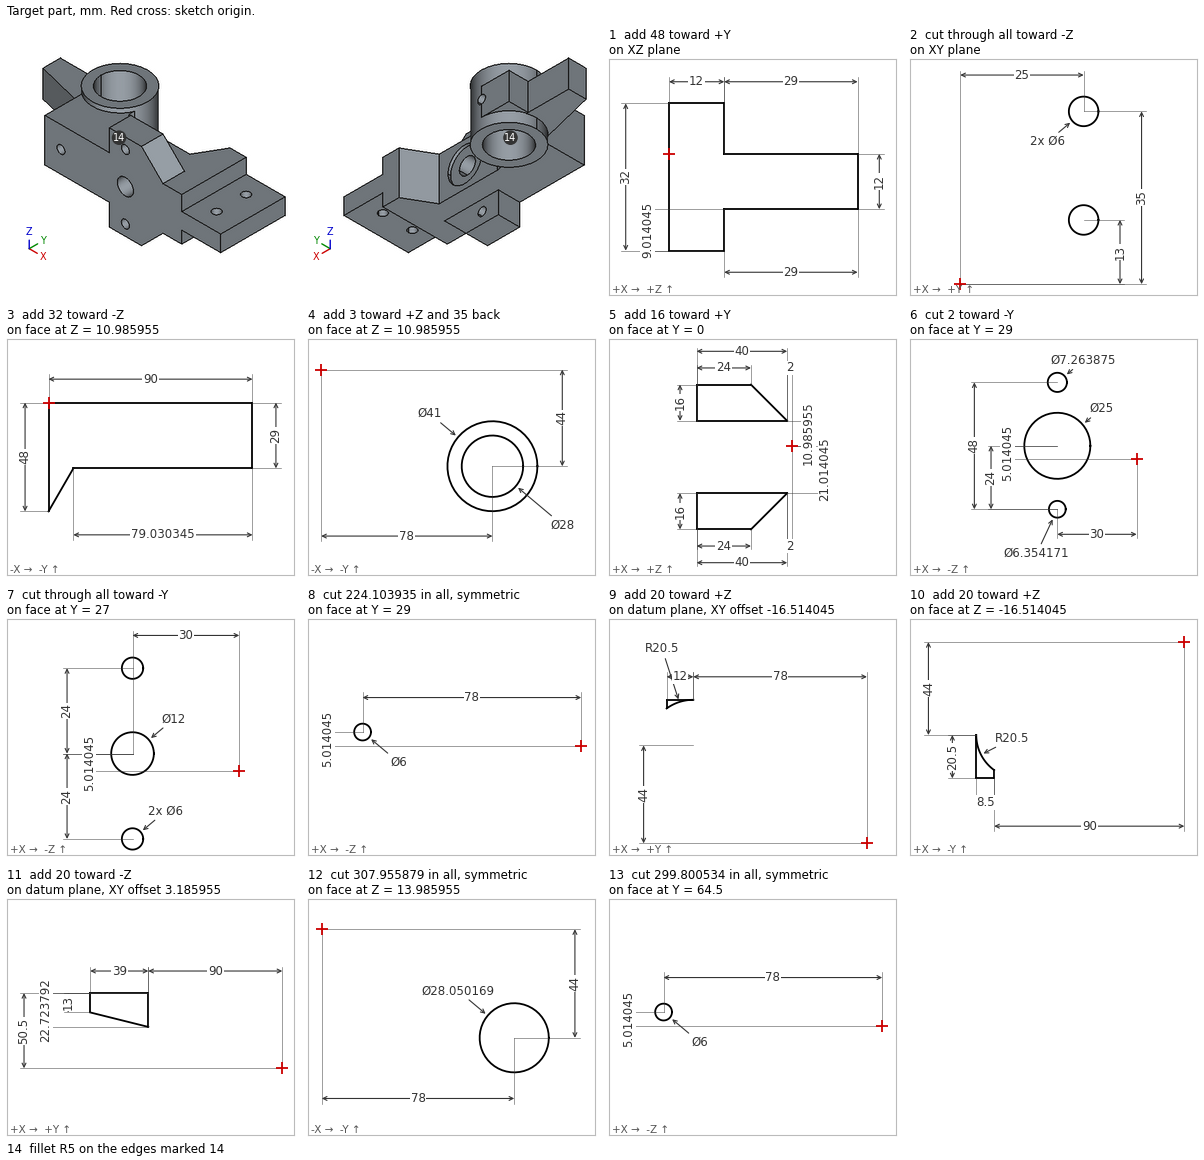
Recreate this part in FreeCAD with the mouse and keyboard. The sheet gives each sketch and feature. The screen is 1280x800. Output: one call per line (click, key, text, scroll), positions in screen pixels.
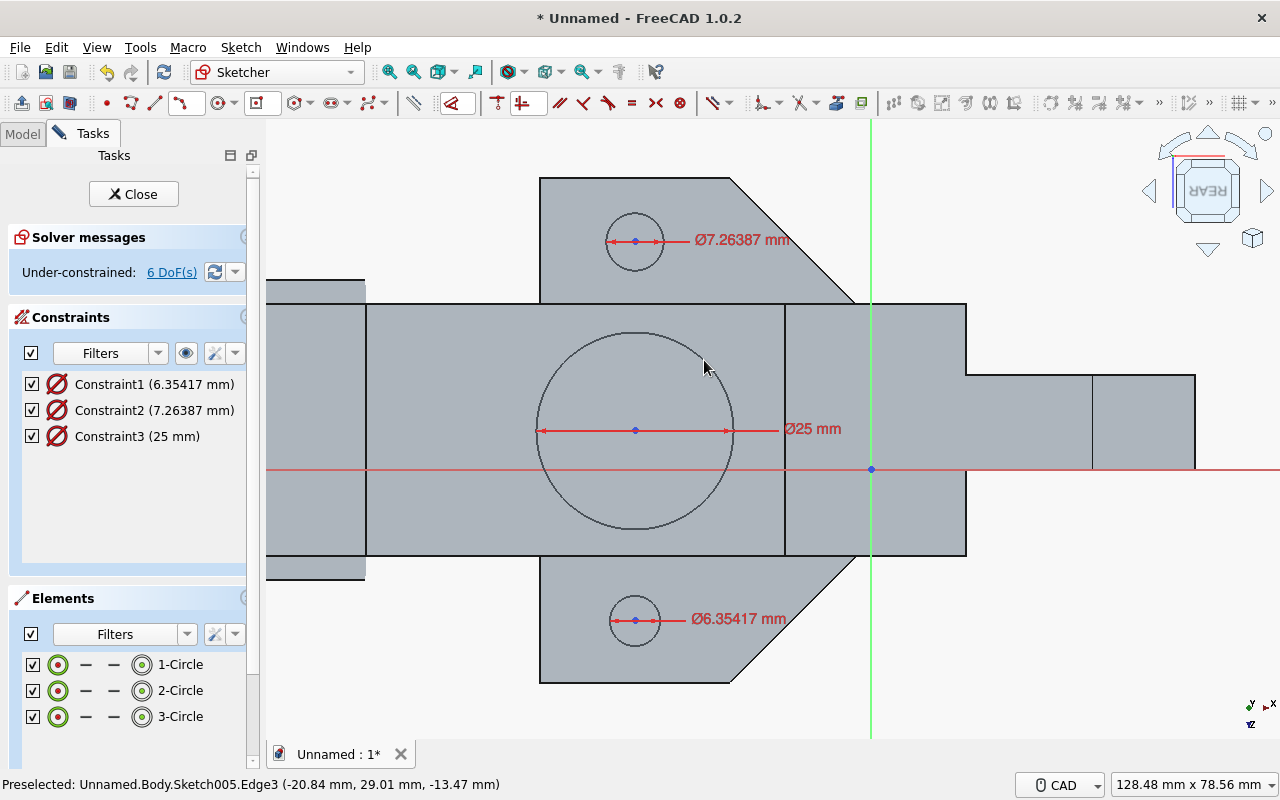
click(635, 621)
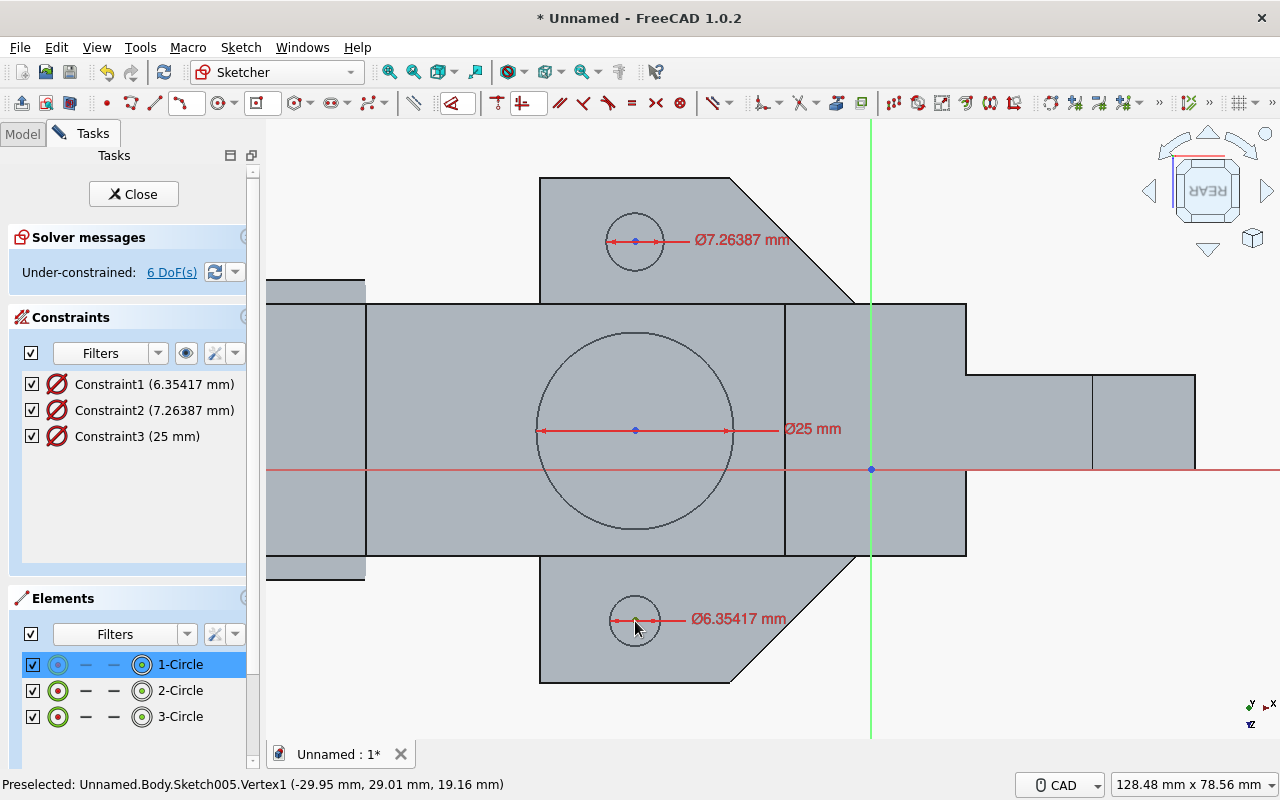
click(635, 242)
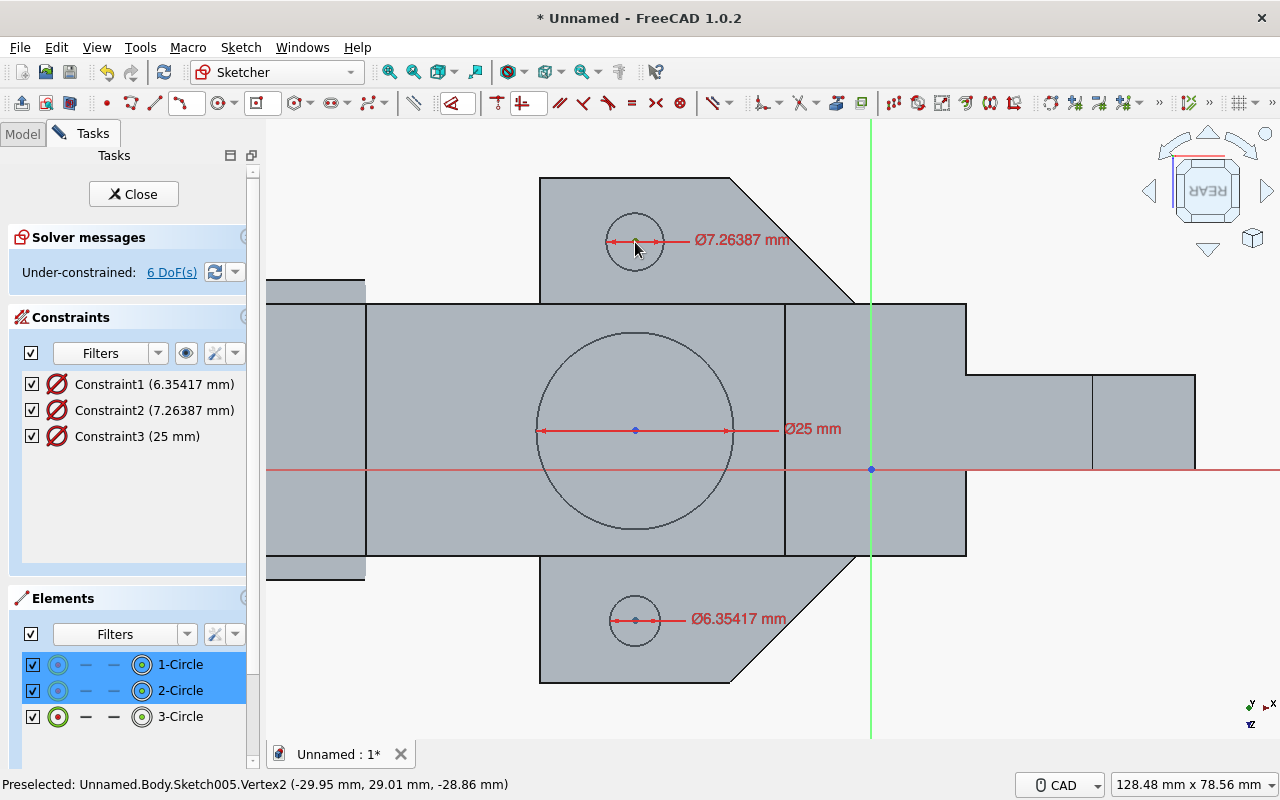
key(v)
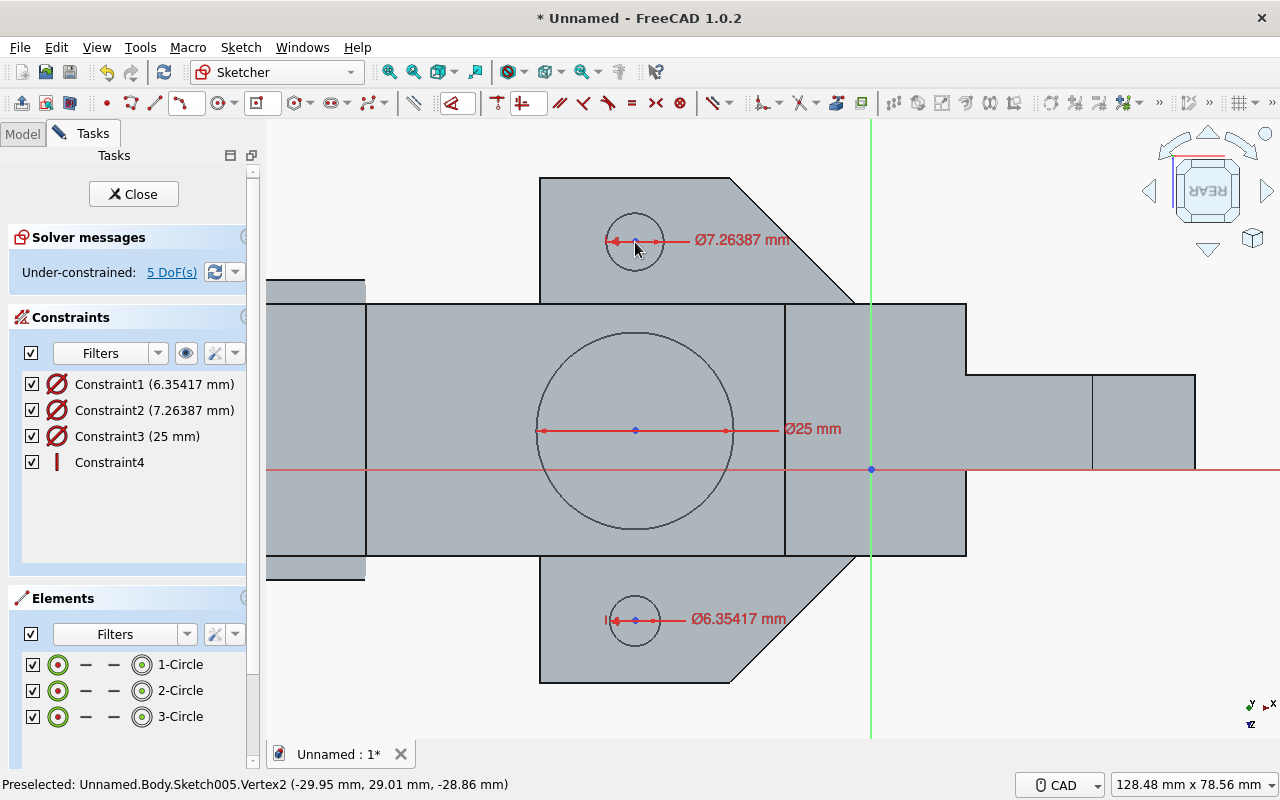
click(635, 621)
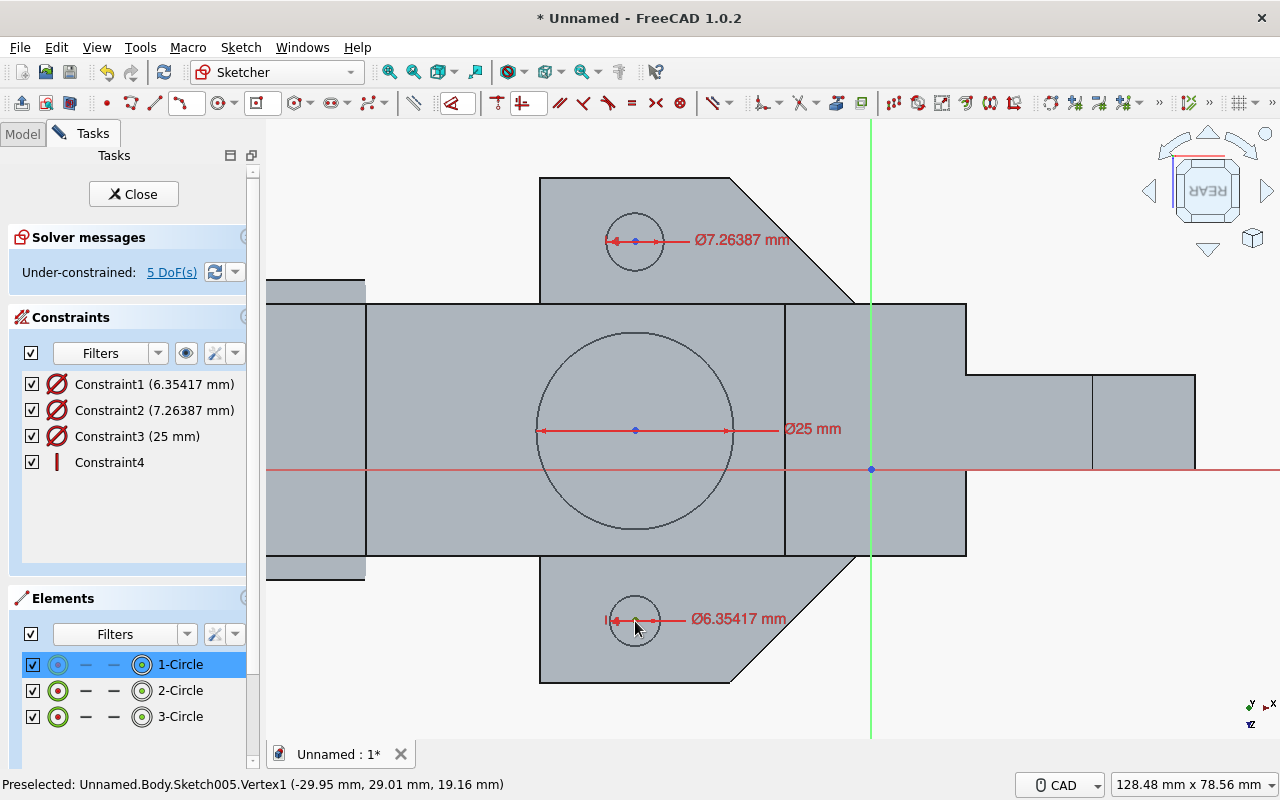
click(635, 431)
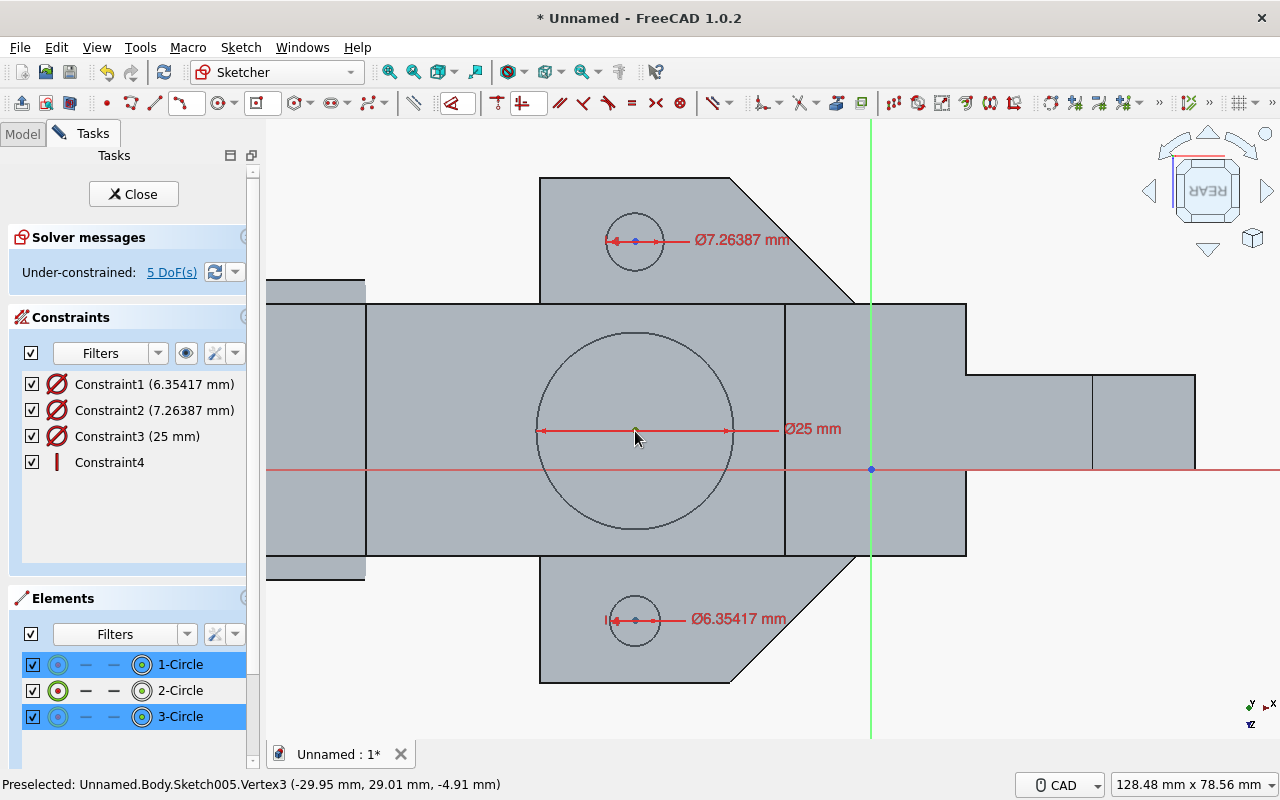
key(v)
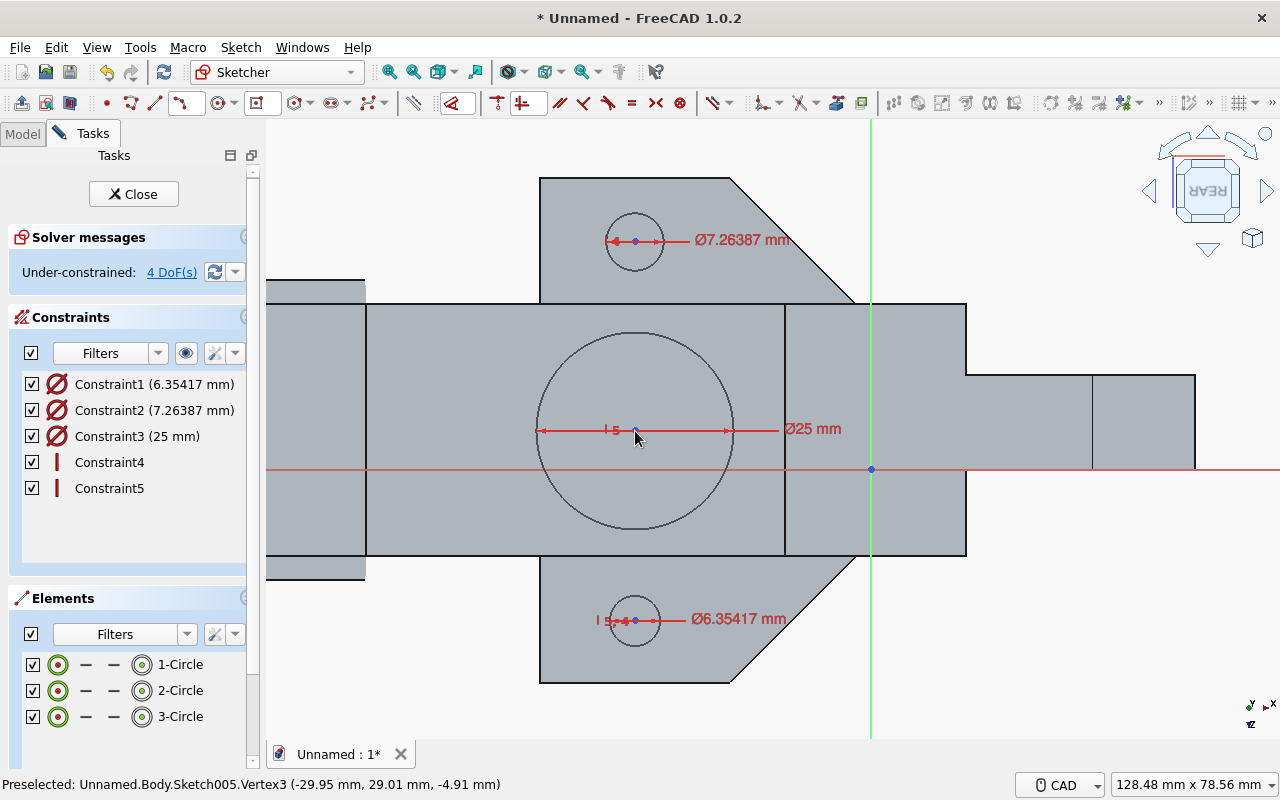
click(635, 621)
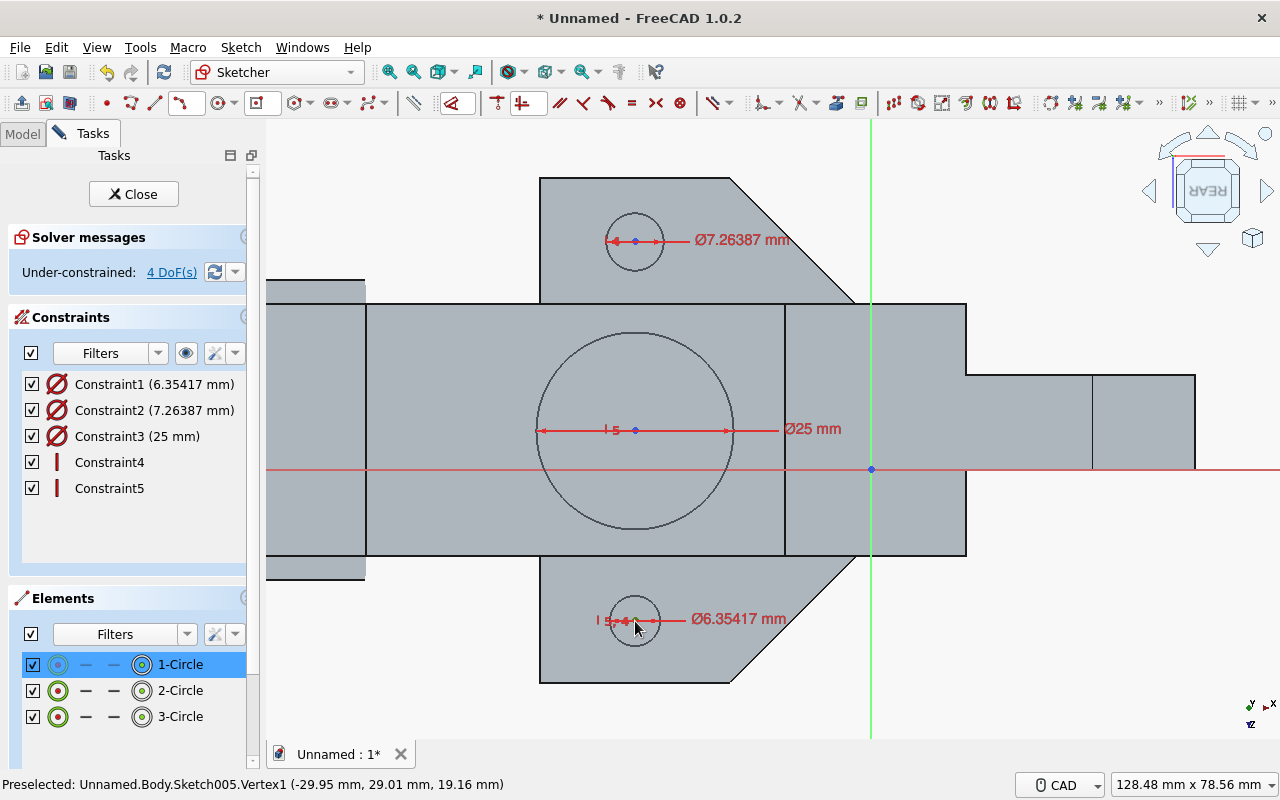
key(l)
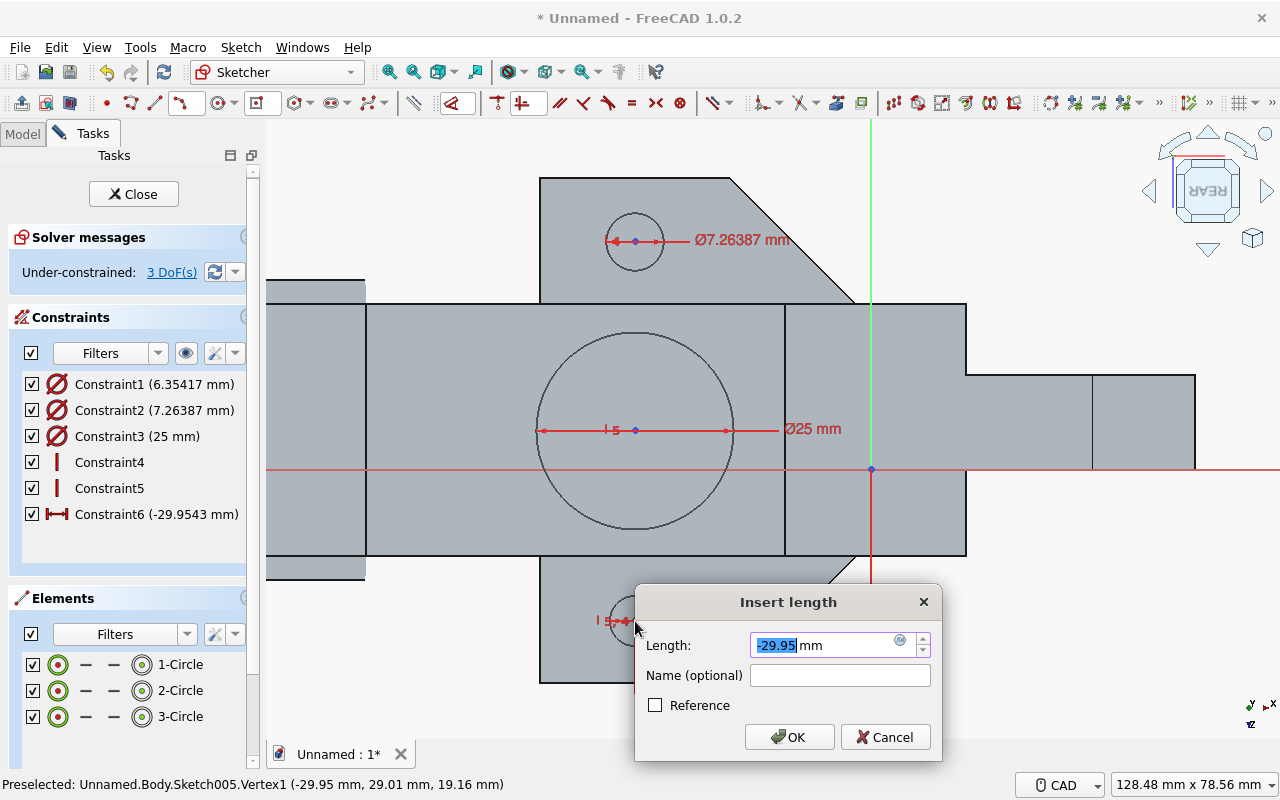
text(-30)
key(Return)